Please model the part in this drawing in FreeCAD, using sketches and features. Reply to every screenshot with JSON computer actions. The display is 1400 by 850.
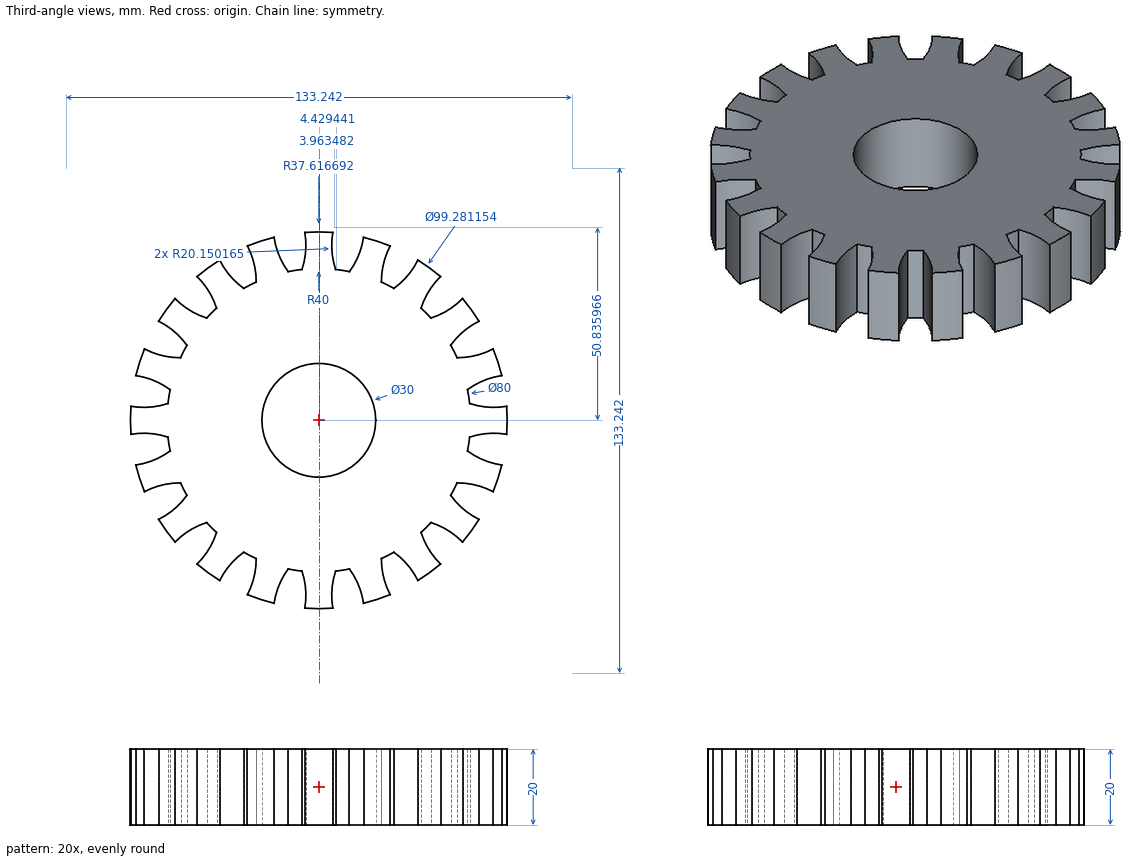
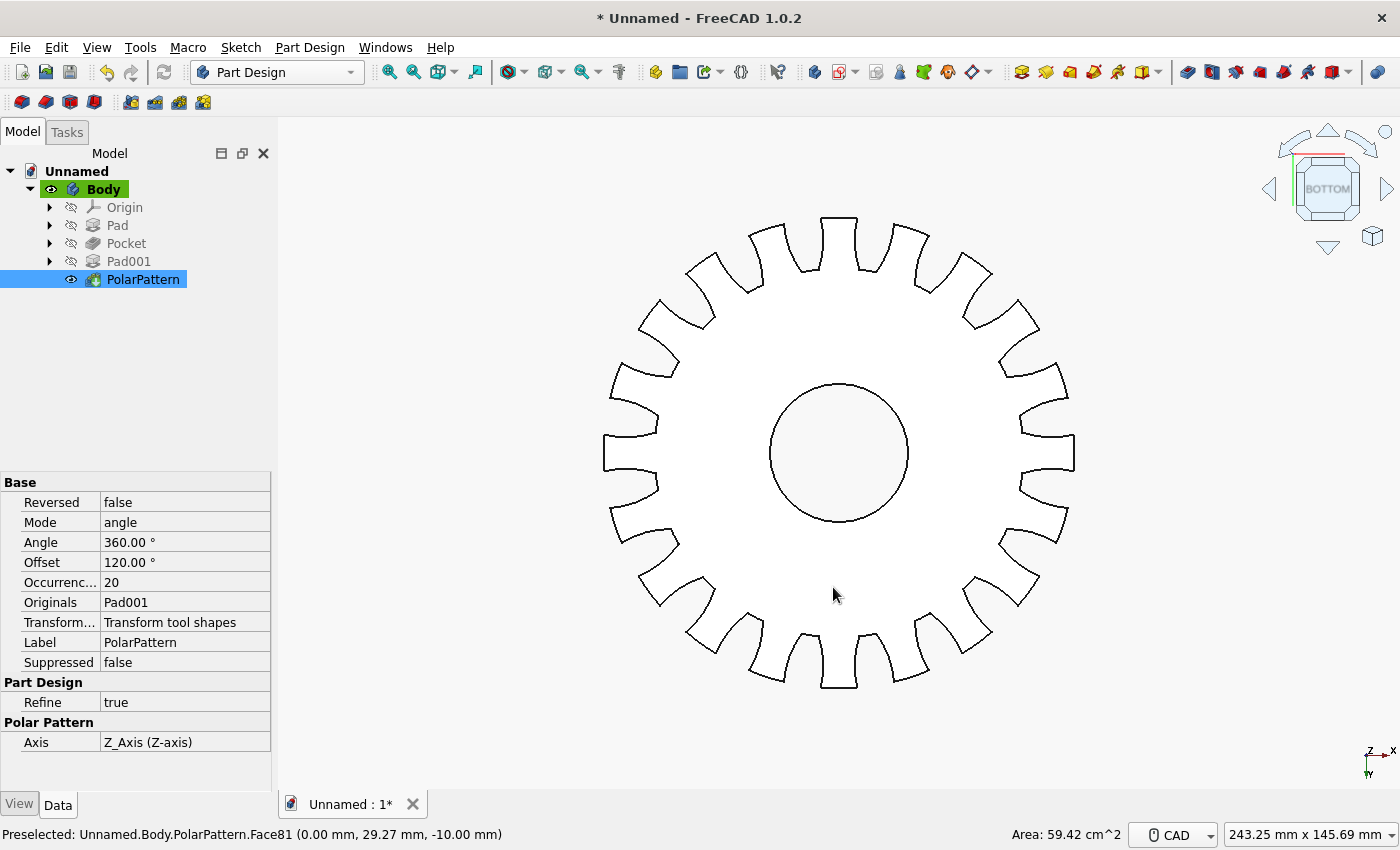
{"action": "left_click", "coordinate": [840, 72]}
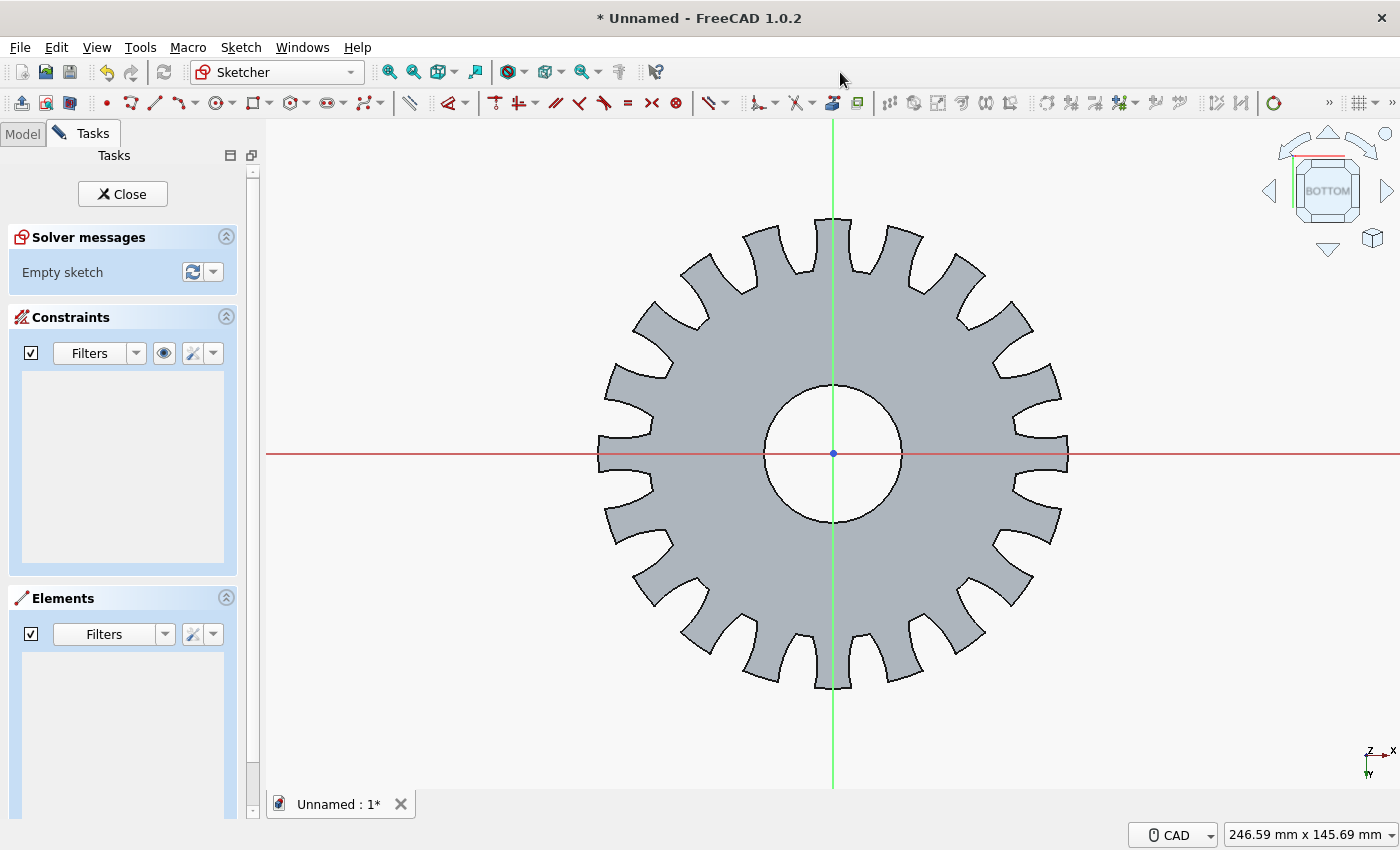
{"action": "scroll", "coordinate": [625, 454], "scroll_direction": "down", "scroll_amount": 2}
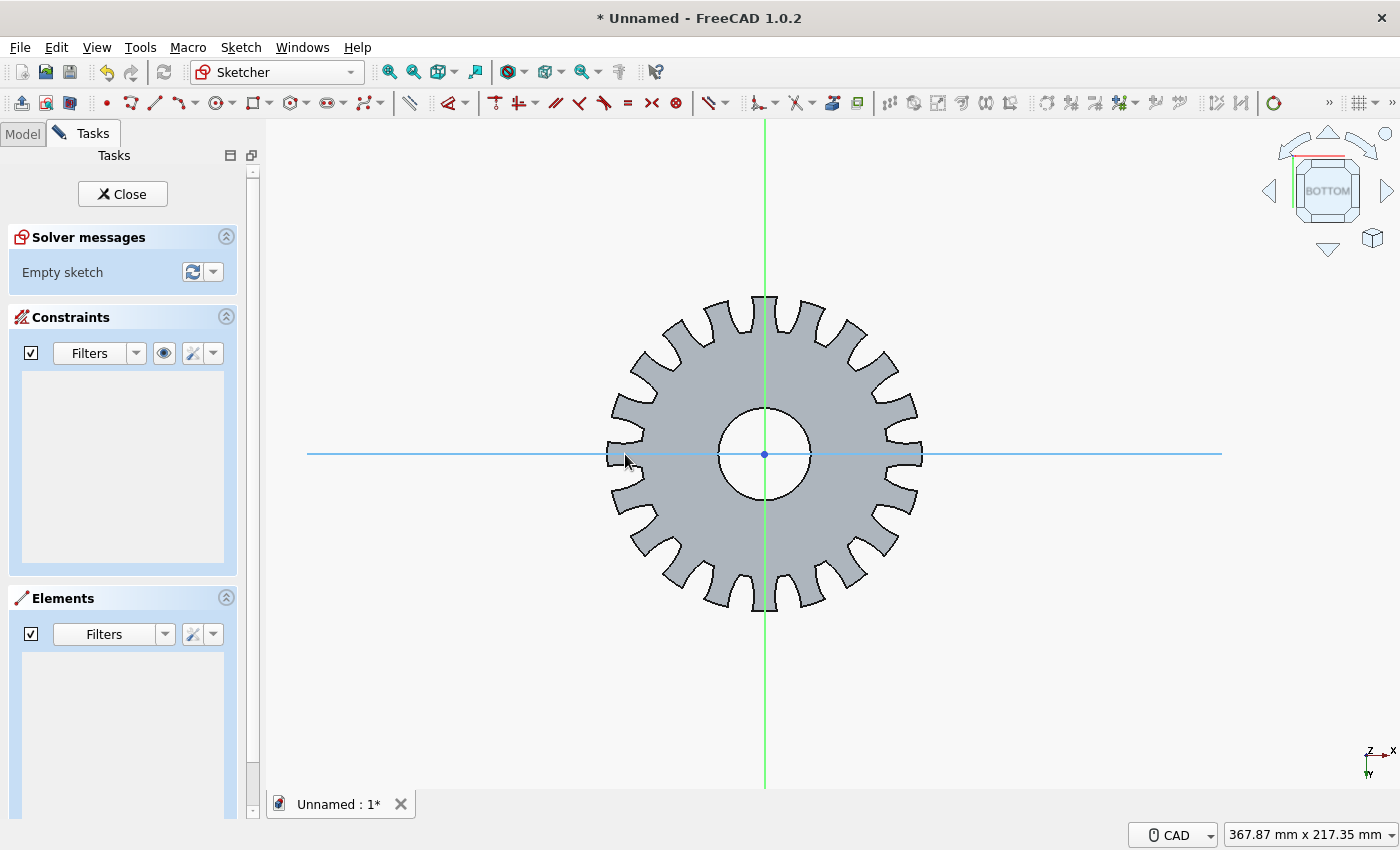
{"action": "key", "text": "g v"}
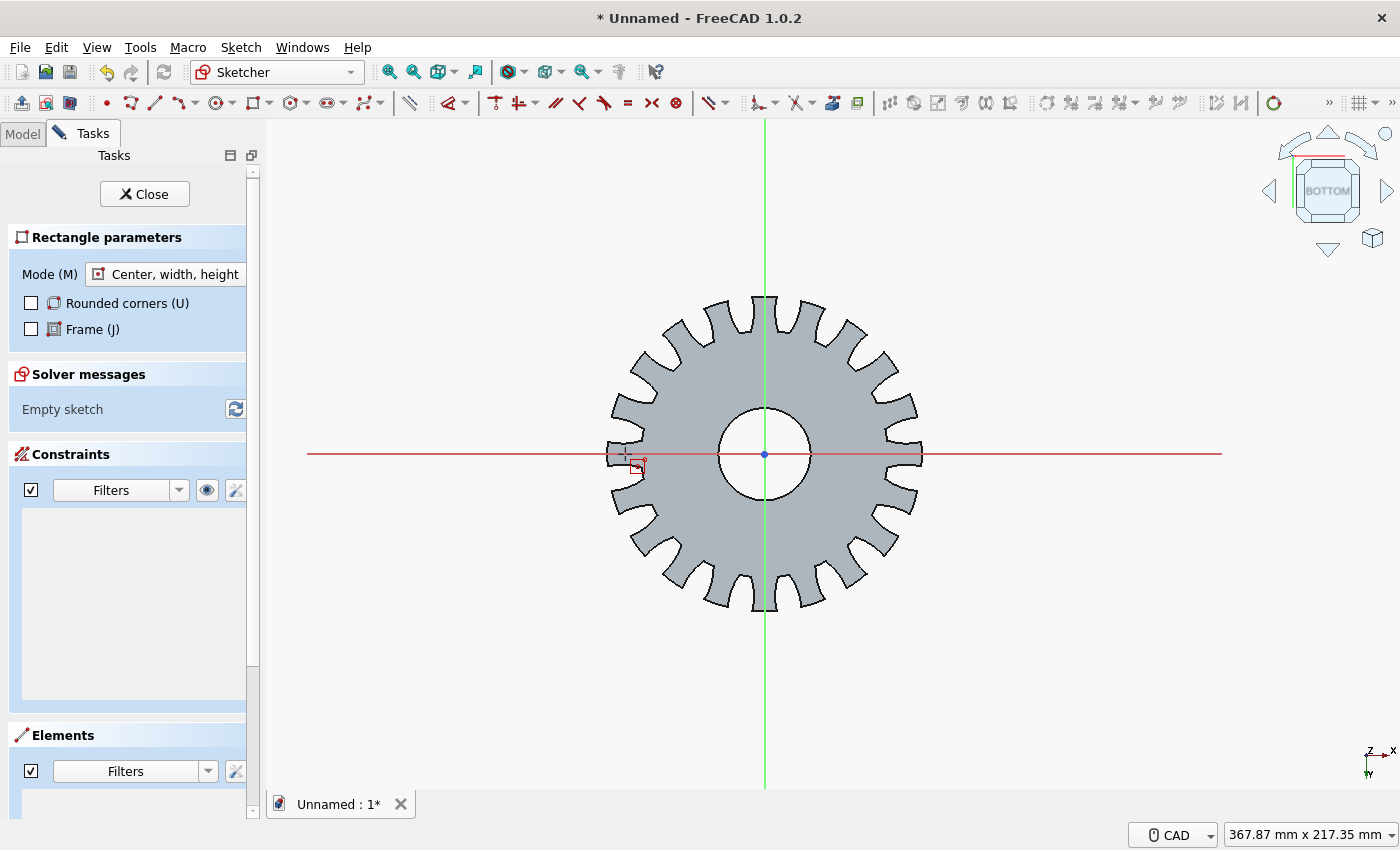
{"action": "left_click", "coordinate": [765, 454]}
{"action": "left_click", "coordinate": [970, 249]}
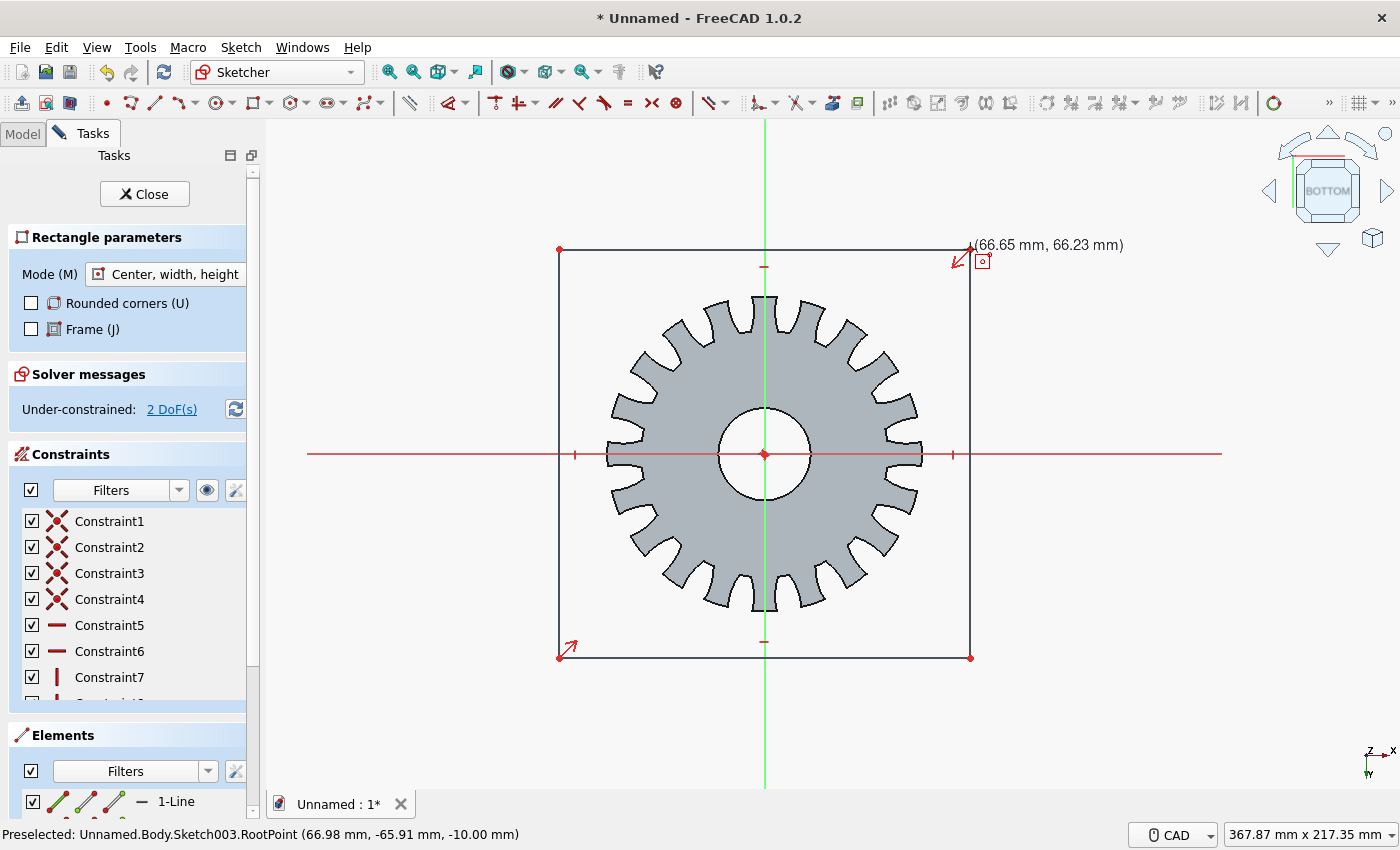
{"action": "left_click", "coordinate": [216, 104]}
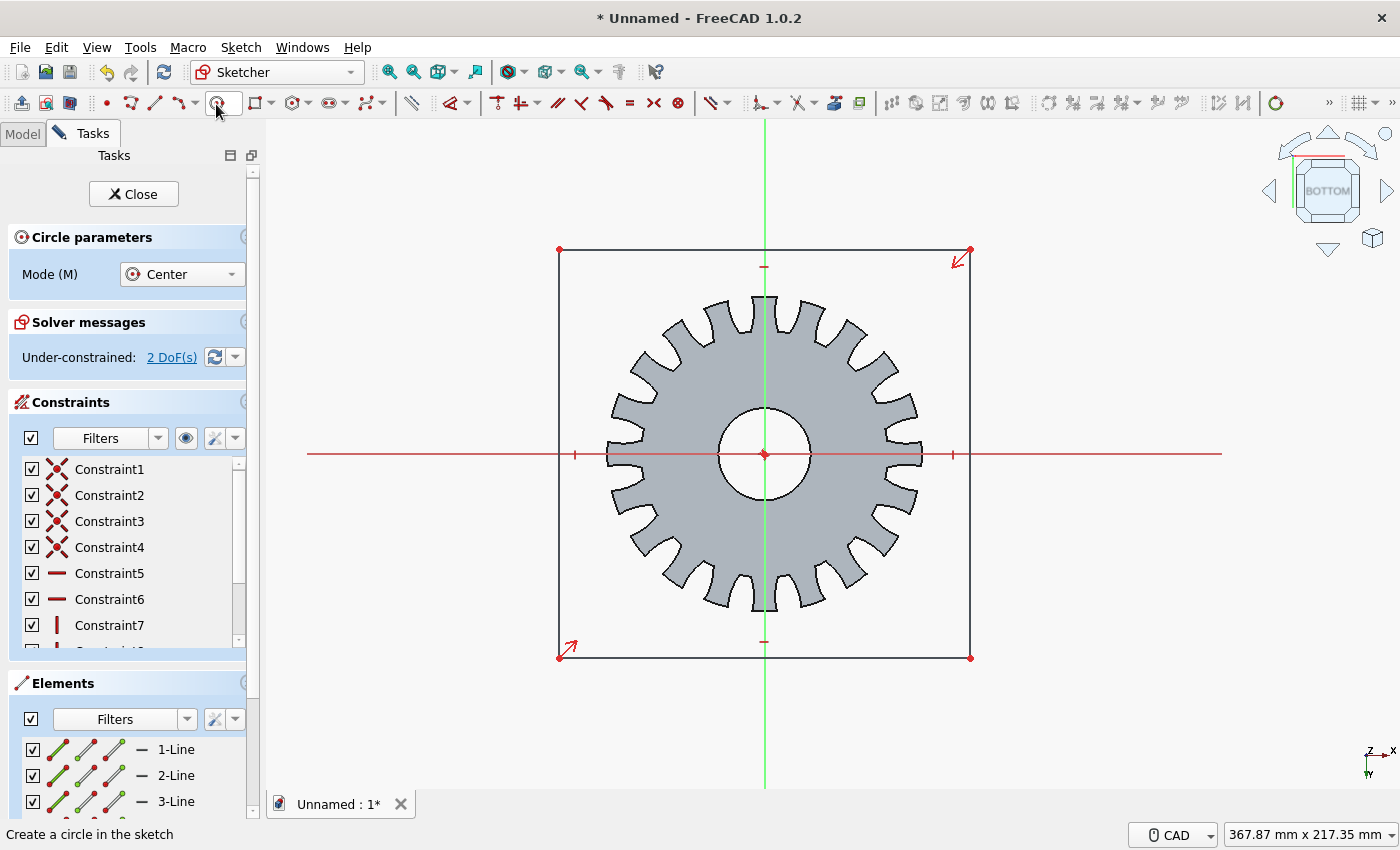
{"action": "left_click", "coordinate": [765, 454]}
{"action": "left_click", "coordinate": [873, 346]}
{"action": "key", "text": "Escape"}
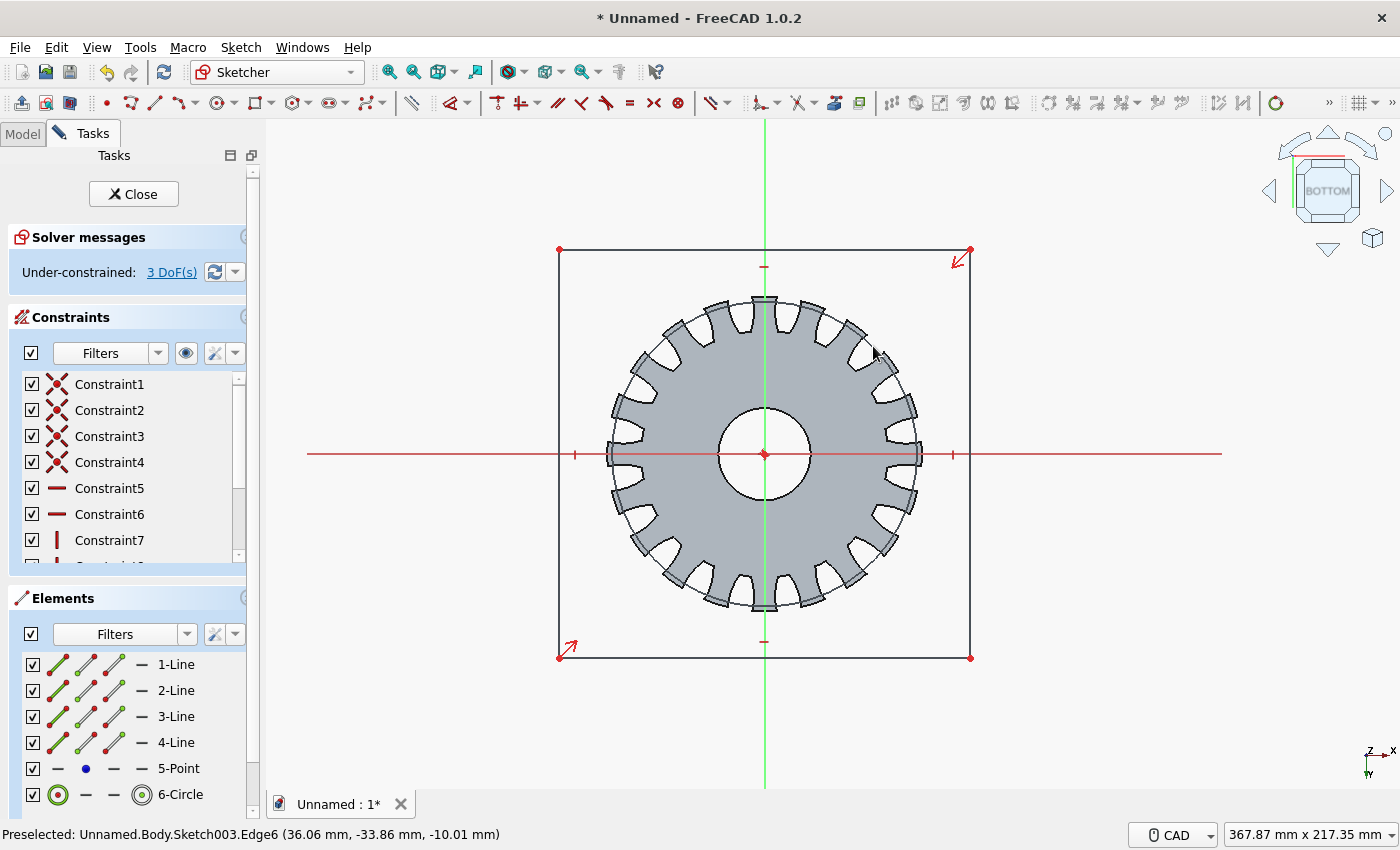
{"action": "left_click", "coordinate": [450, 104]}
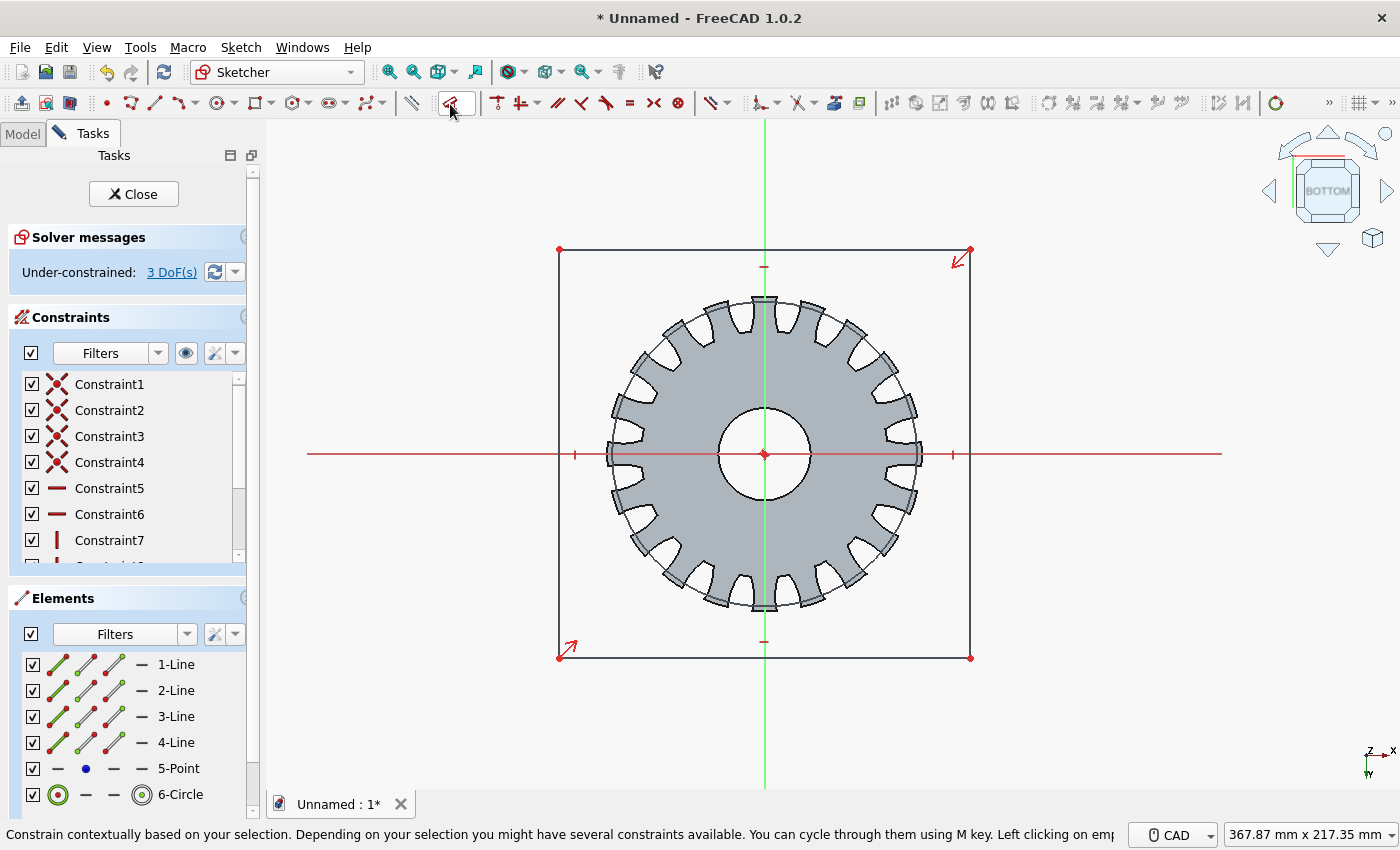
{"action": "left_click", "coordinate": [872, 346]}
{"action": "left_click", "coordinate": [895, 323]}